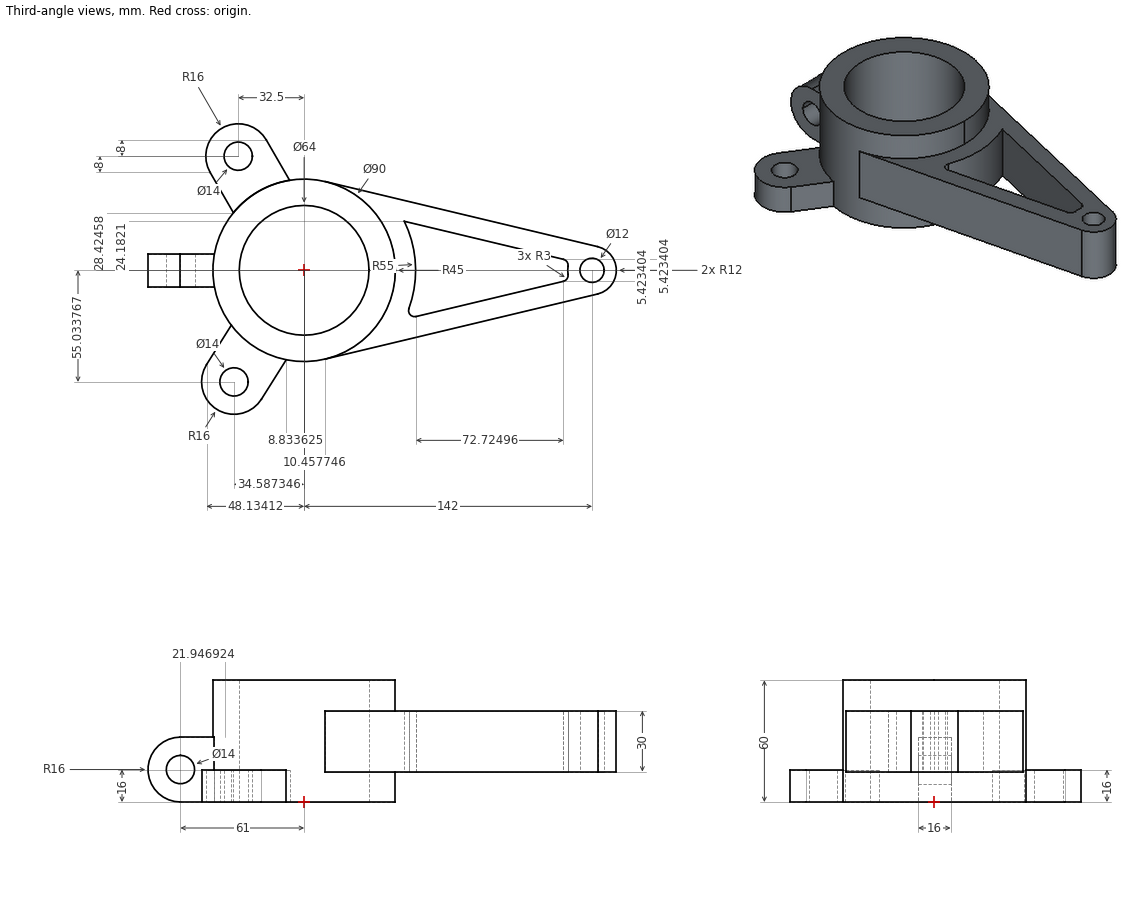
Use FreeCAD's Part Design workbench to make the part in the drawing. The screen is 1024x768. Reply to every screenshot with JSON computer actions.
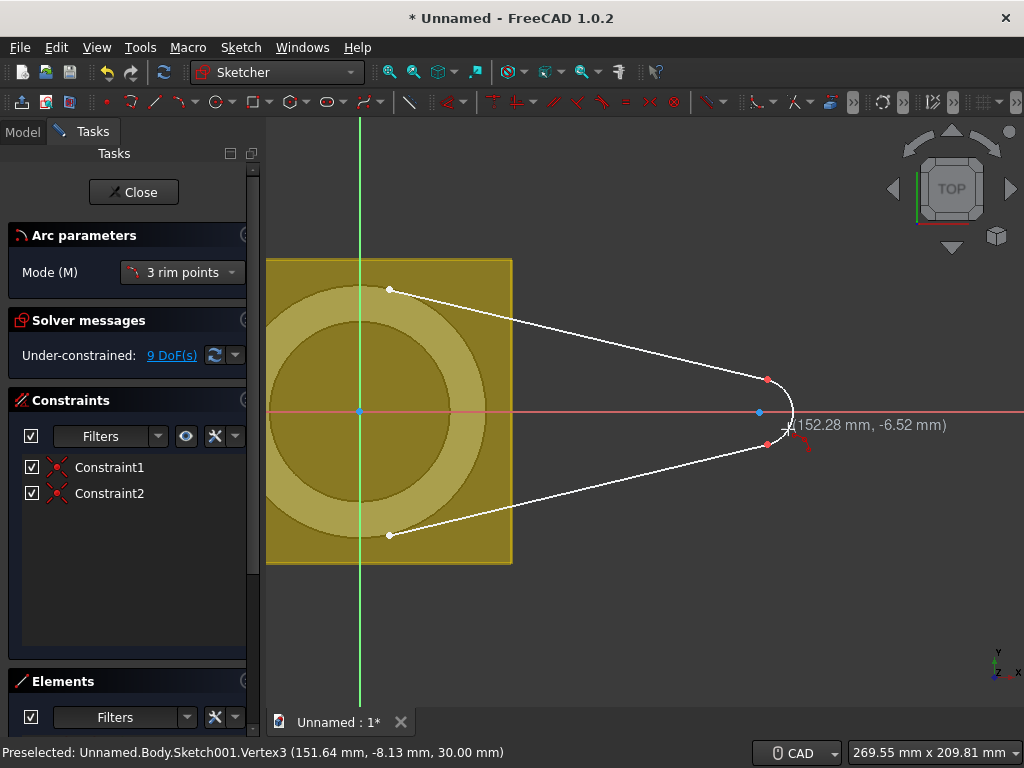
{"action": "left_click", "coordinate": [389, 290]}
{"action": "left_click", "coordinate": [389, 536]}
{"action": "left_click", "coordinate": [482, 445]}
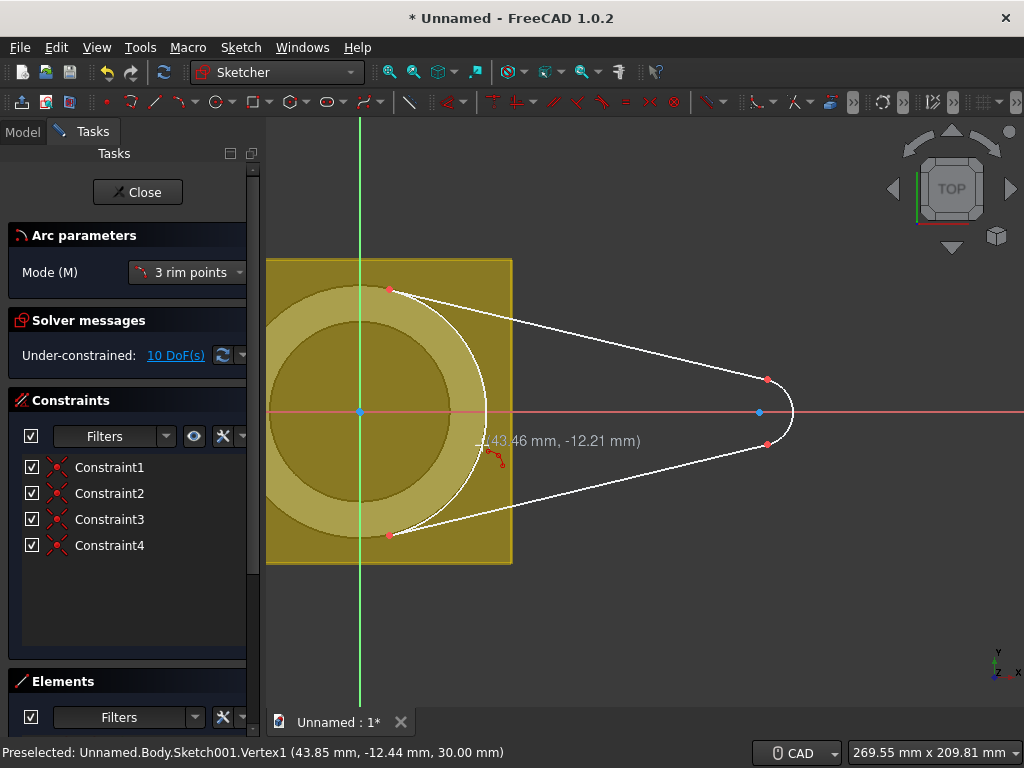
{"action": "left_click", "coordinate": [156, 102]}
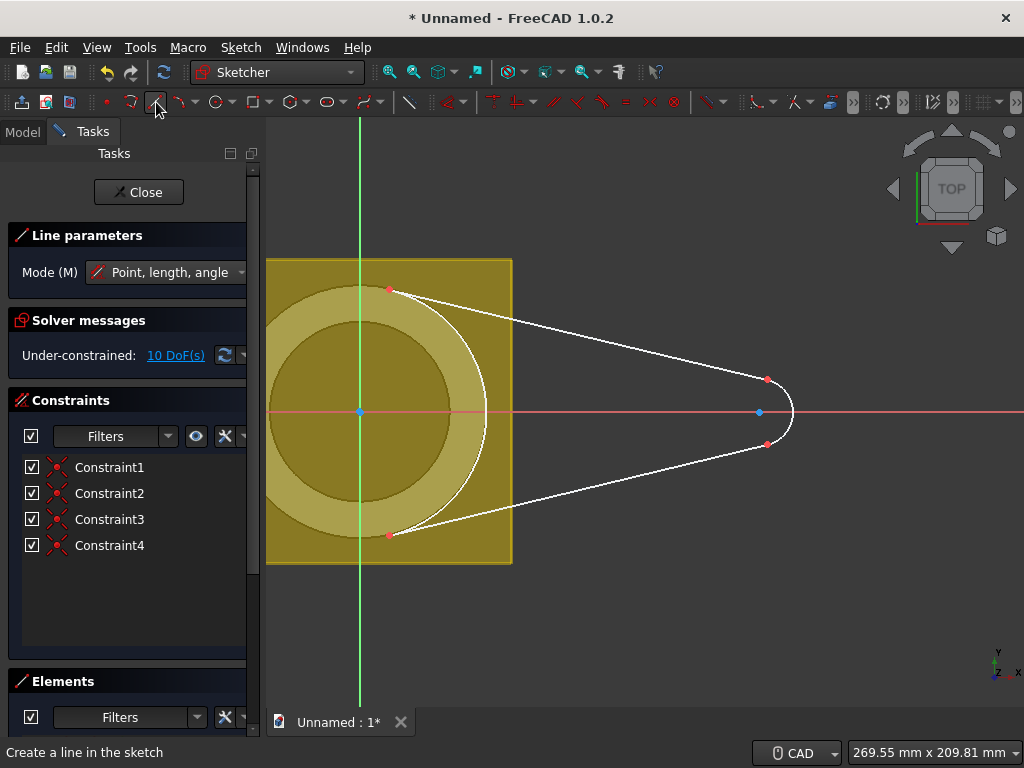
{"action": "left_click", "coordinate": [719, 427]}
{"action": "left_click", "coordinate": [515, 476]}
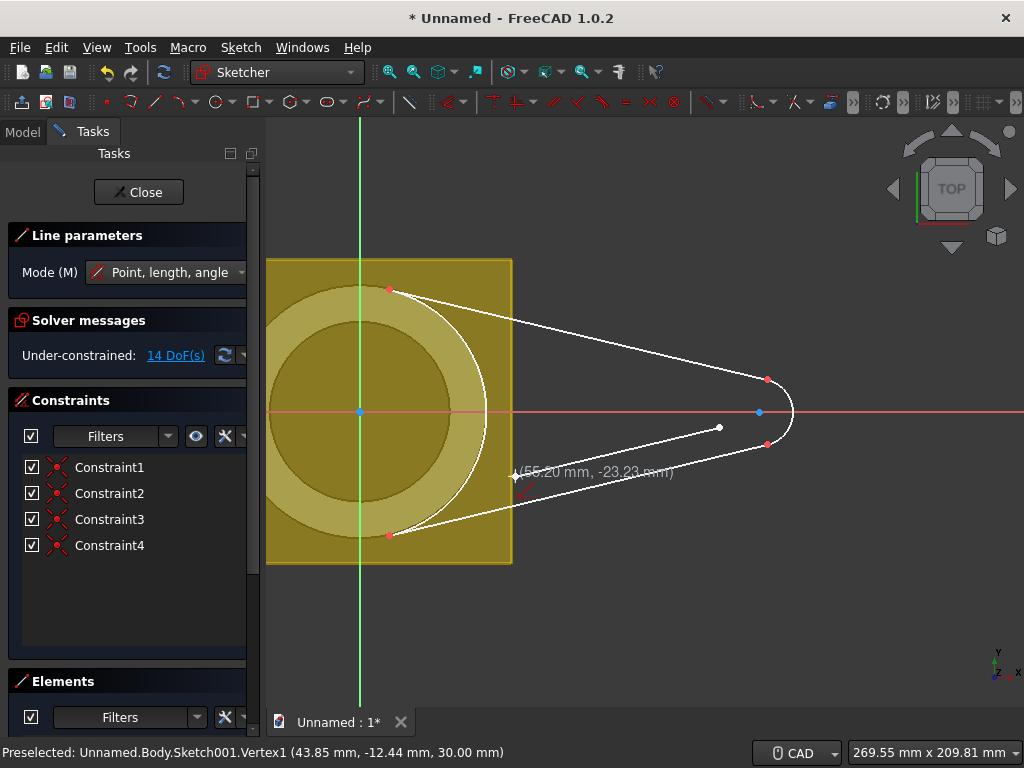
{"action": "left_click", "coordinate": [499, 344]}
{"action": "left_click", "coordinate": [719, 396]}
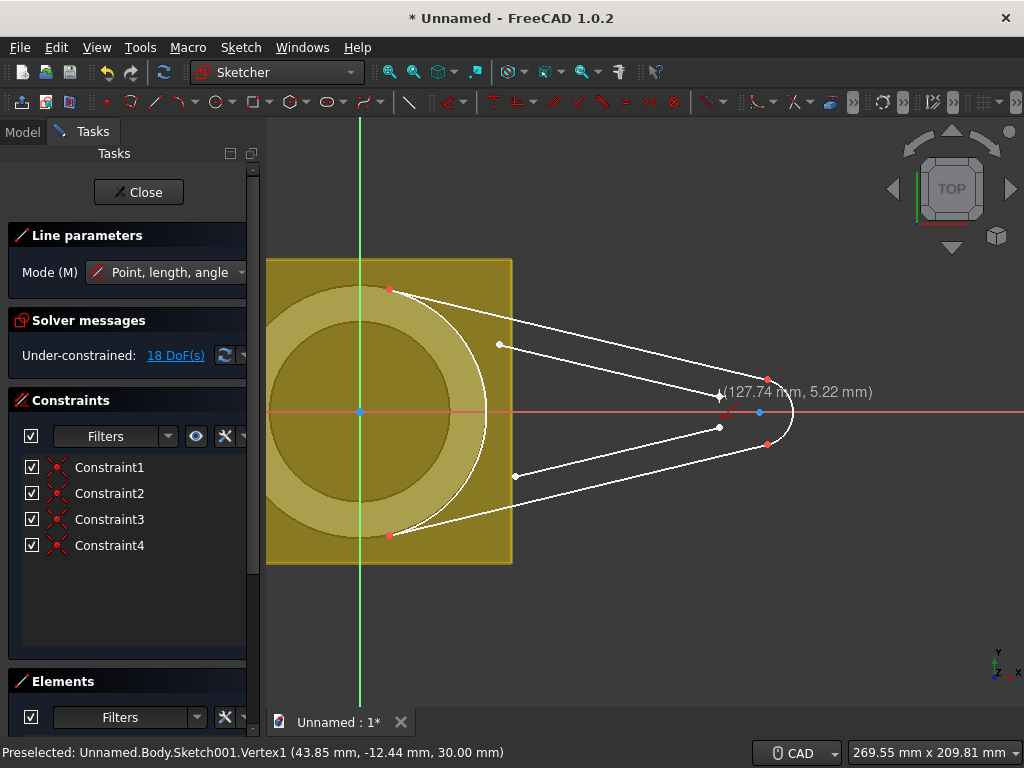
{"action": "key", "text": "g 3 a"}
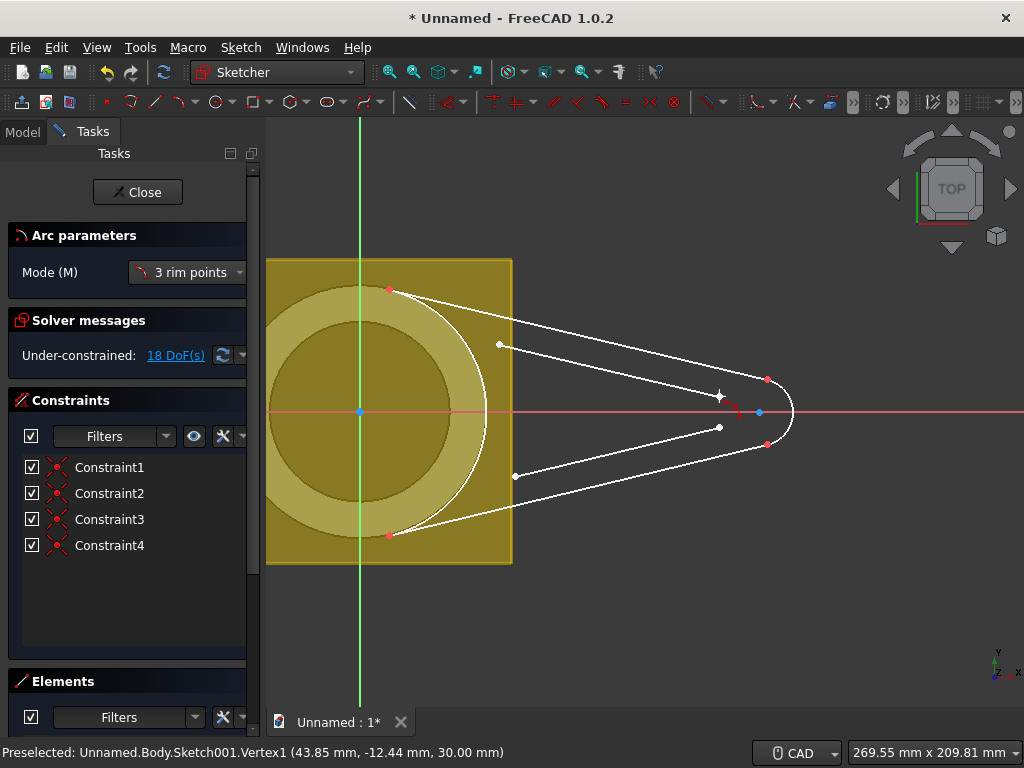
{"action": "left_click", "coordinate": [515, 477]}
{"action": "left_click", "coordinate": [505, 465]}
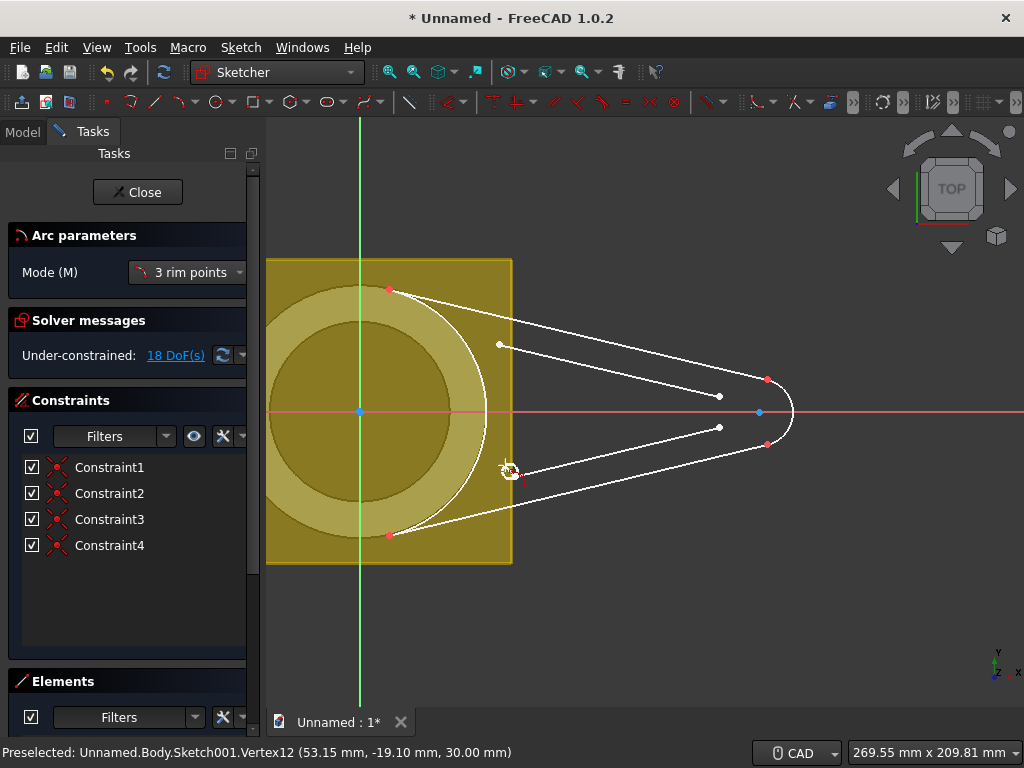
{"action": "scroll", "coordinate": [507, 473], "scroll_direction": "up", "scroll_amount": 7}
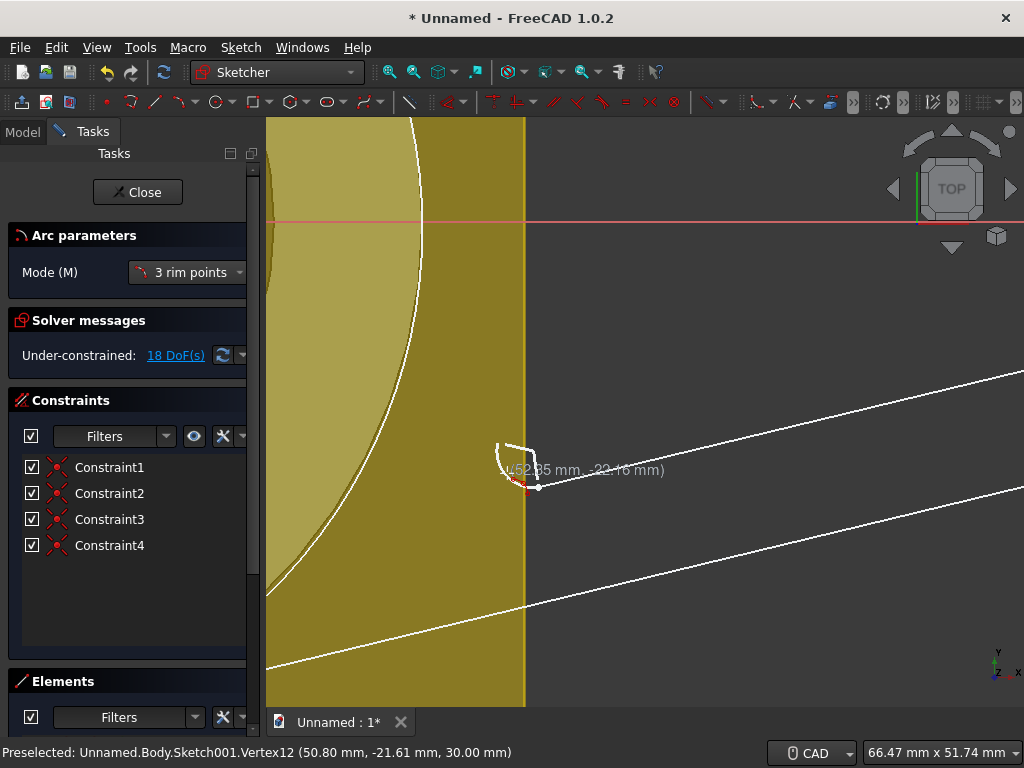
{"action": "left_click", "coordinate": [505, 472]}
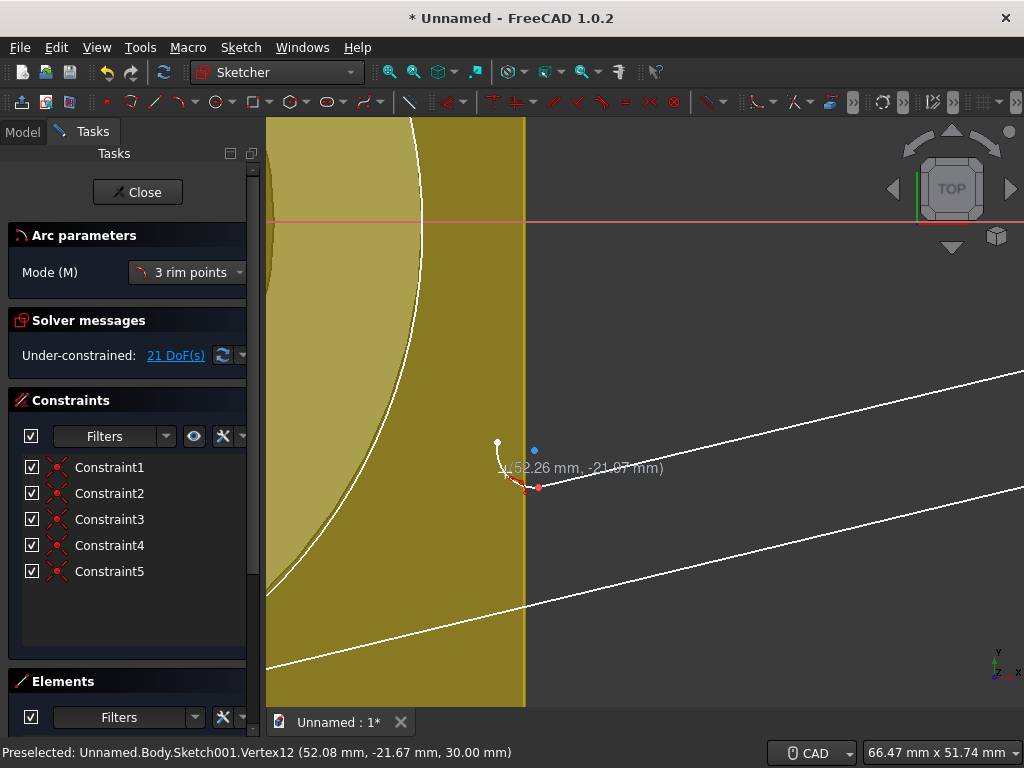
{"action": "left_click", "coordinate": [498, 443]}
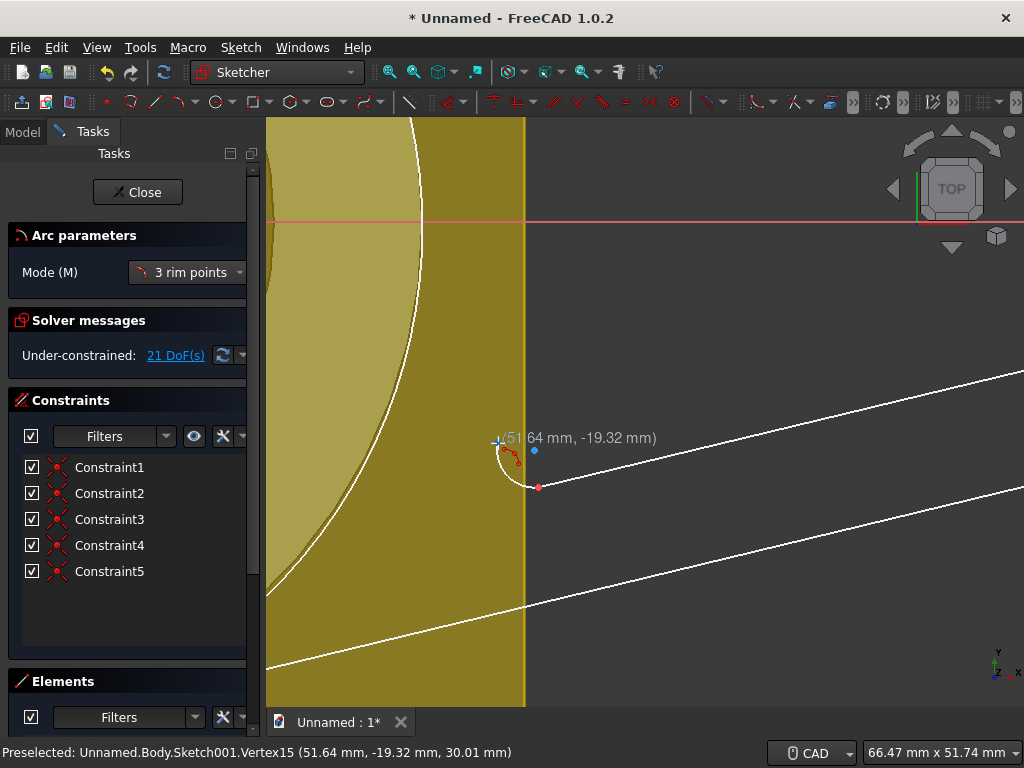
{"action": "scroll", "coordinate": [508, 474], "scroll_direction": "down", "scroll_amount": 7}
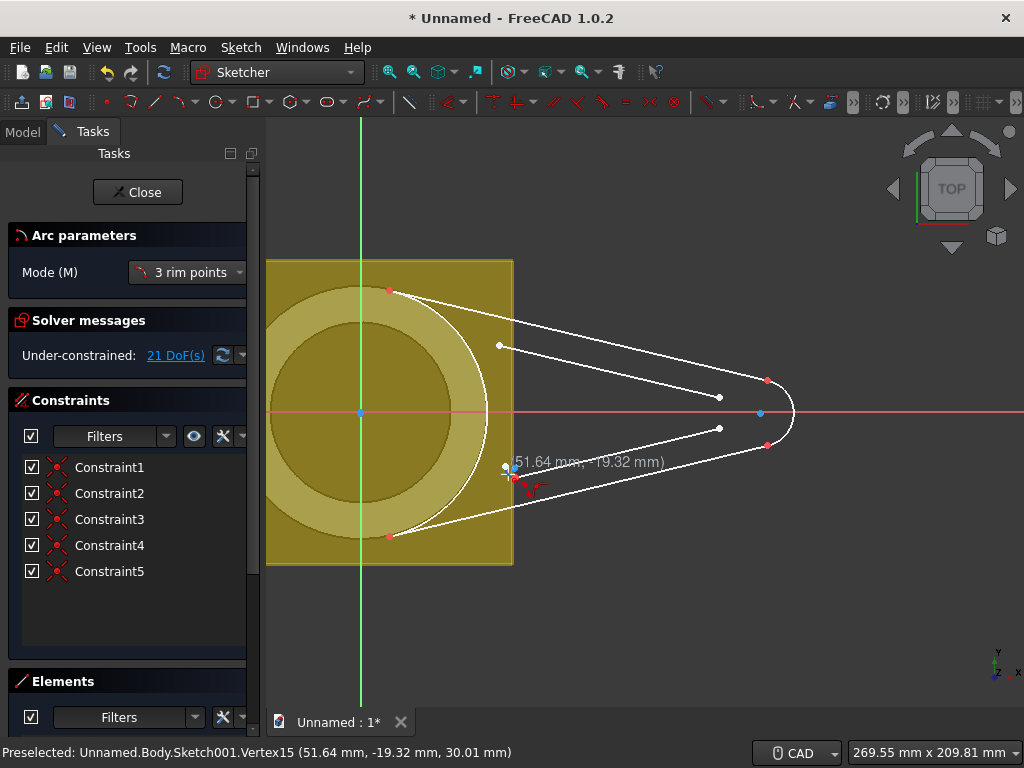
{"action": "left_click", "coordinate": [500, 346]}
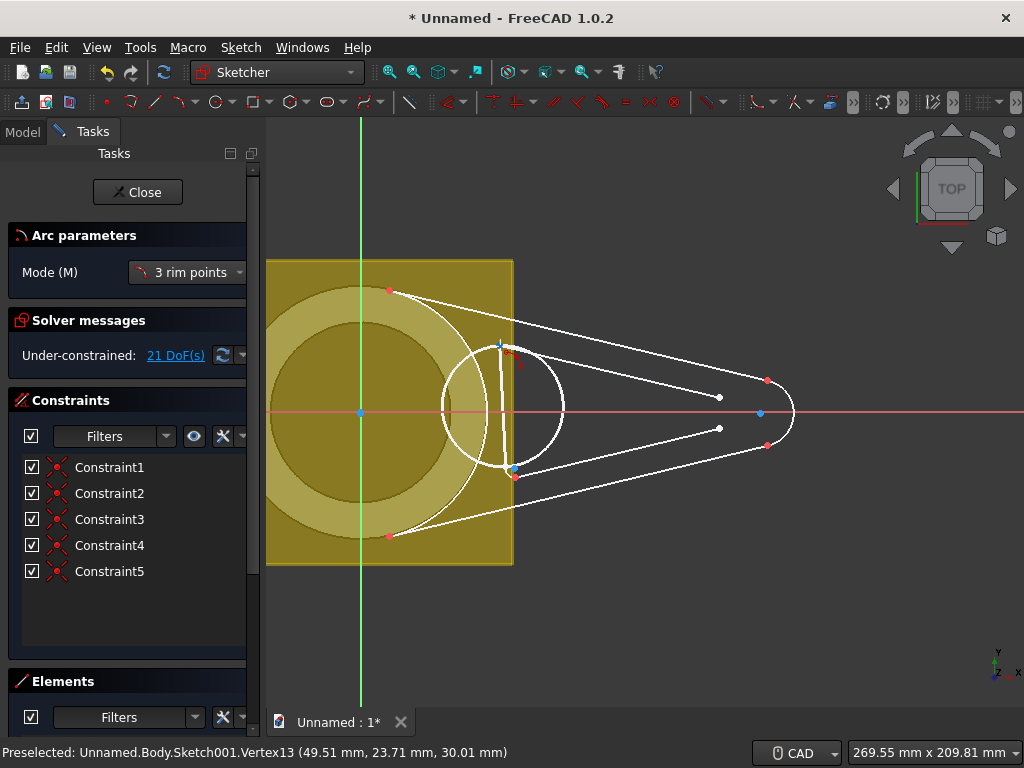
{"action": "scroll", "coordinate": [514, 392], "scroll_direction": "up", "scroll_amount": 2}